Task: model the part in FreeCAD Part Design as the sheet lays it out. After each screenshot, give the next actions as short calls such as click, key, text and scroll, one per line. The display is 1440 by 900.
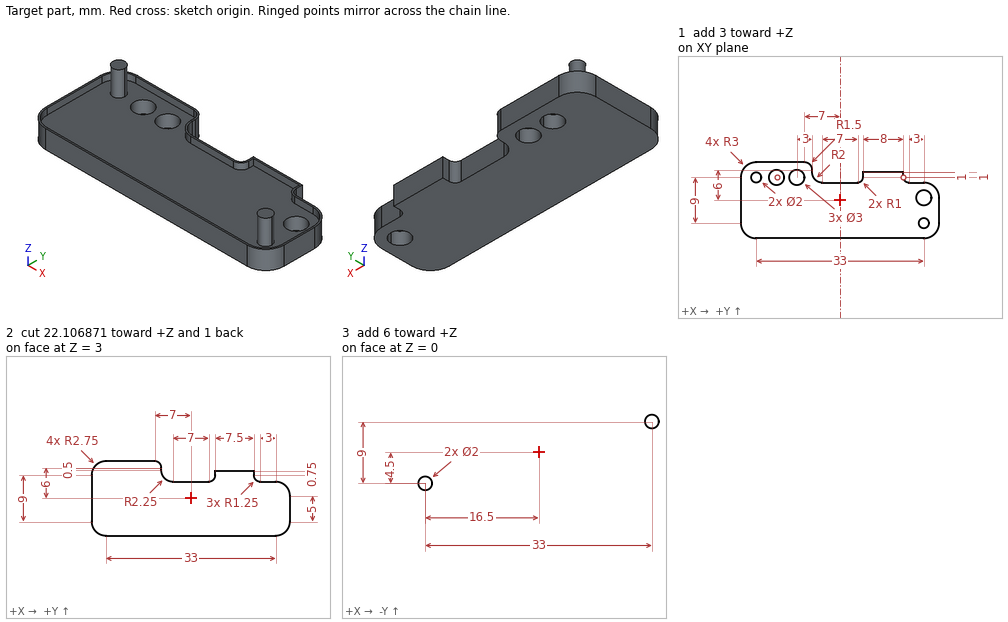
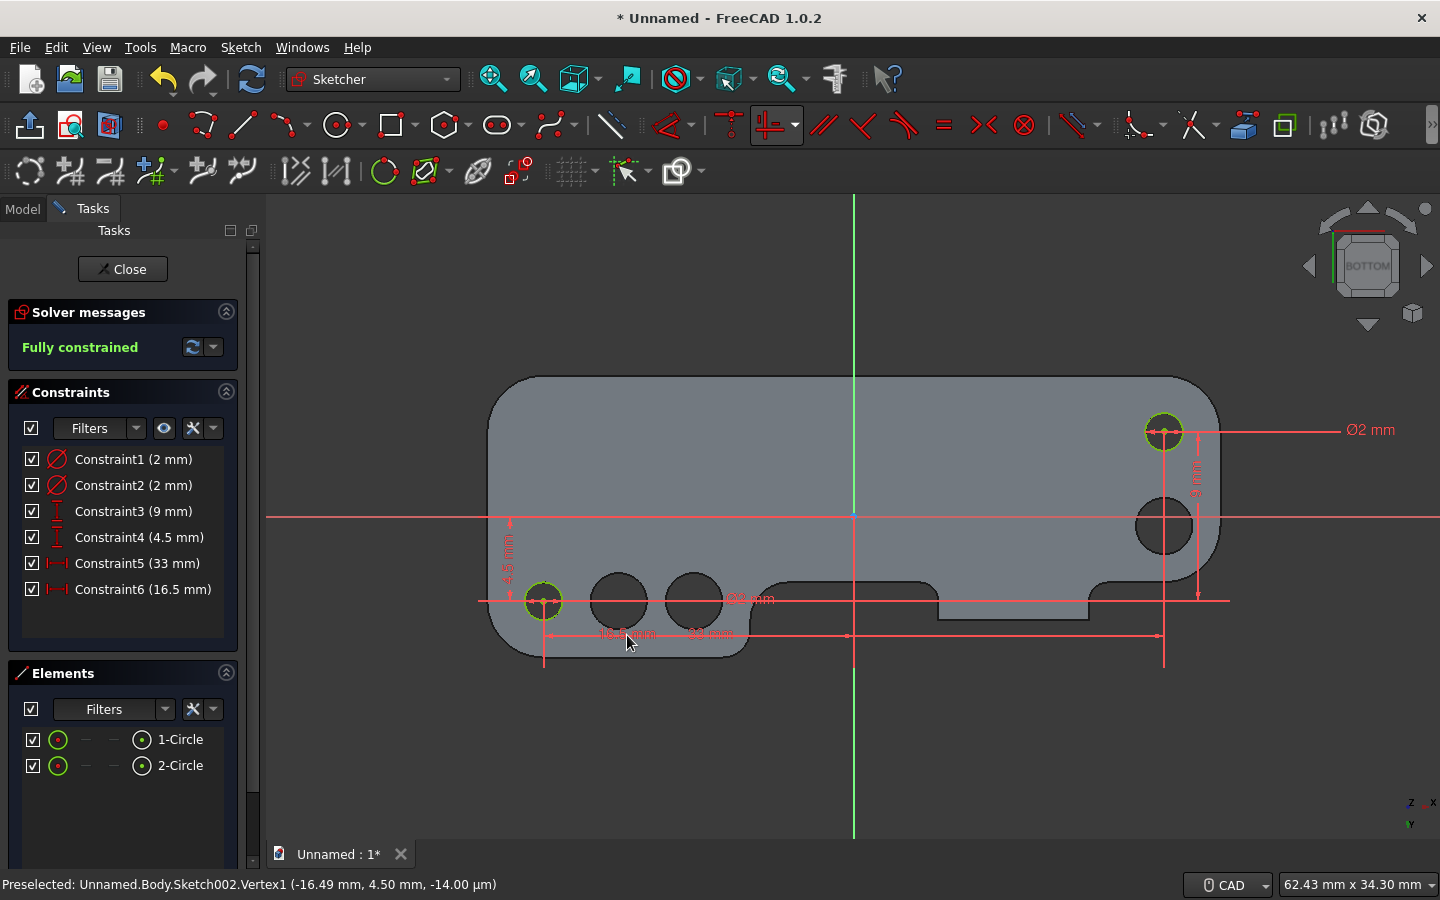
click(123, 269)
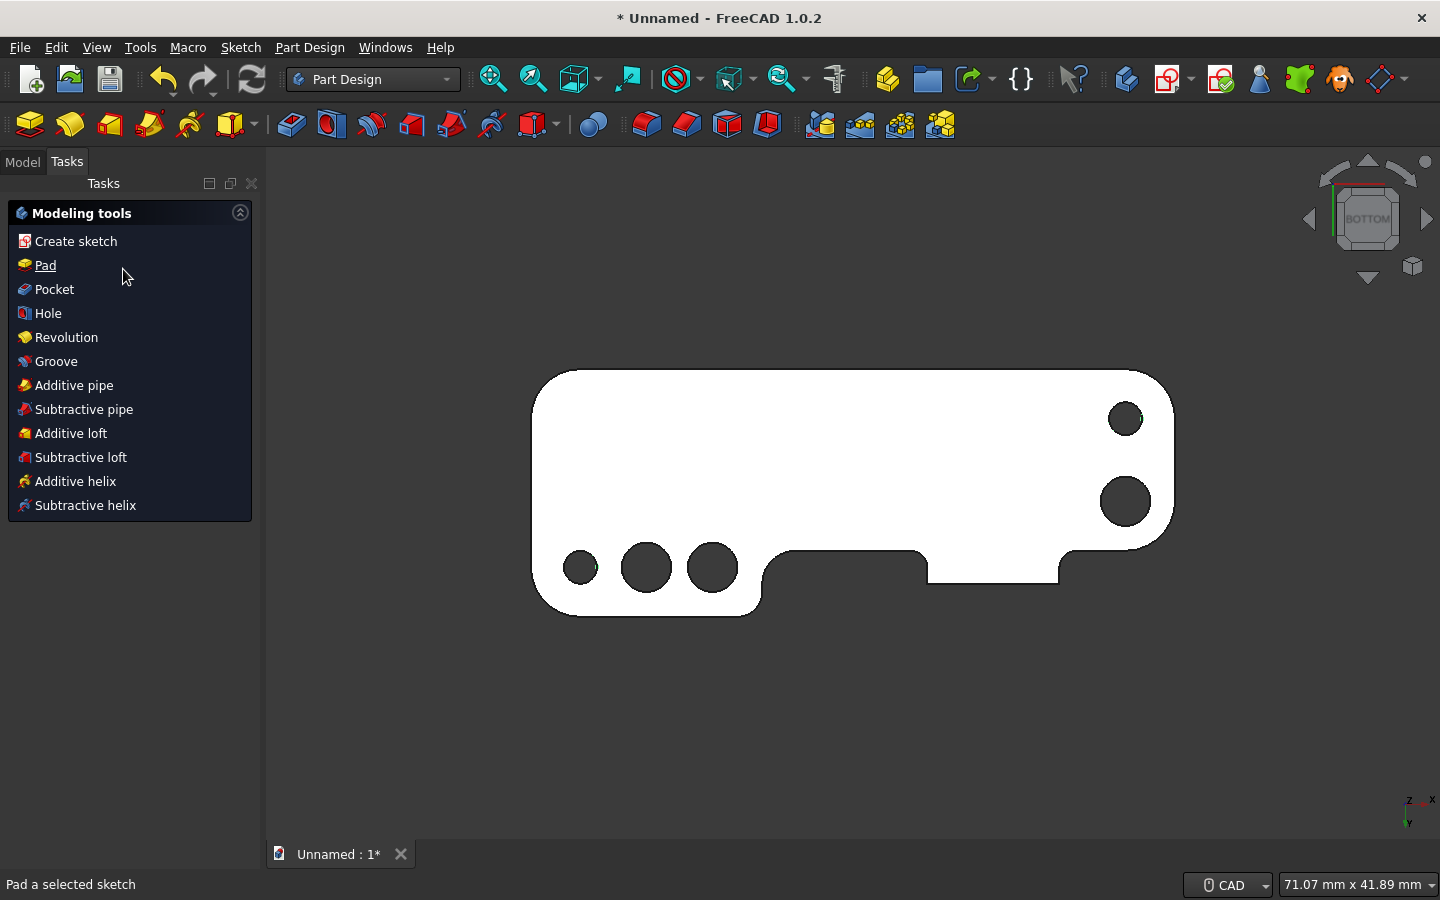
click(30, 124)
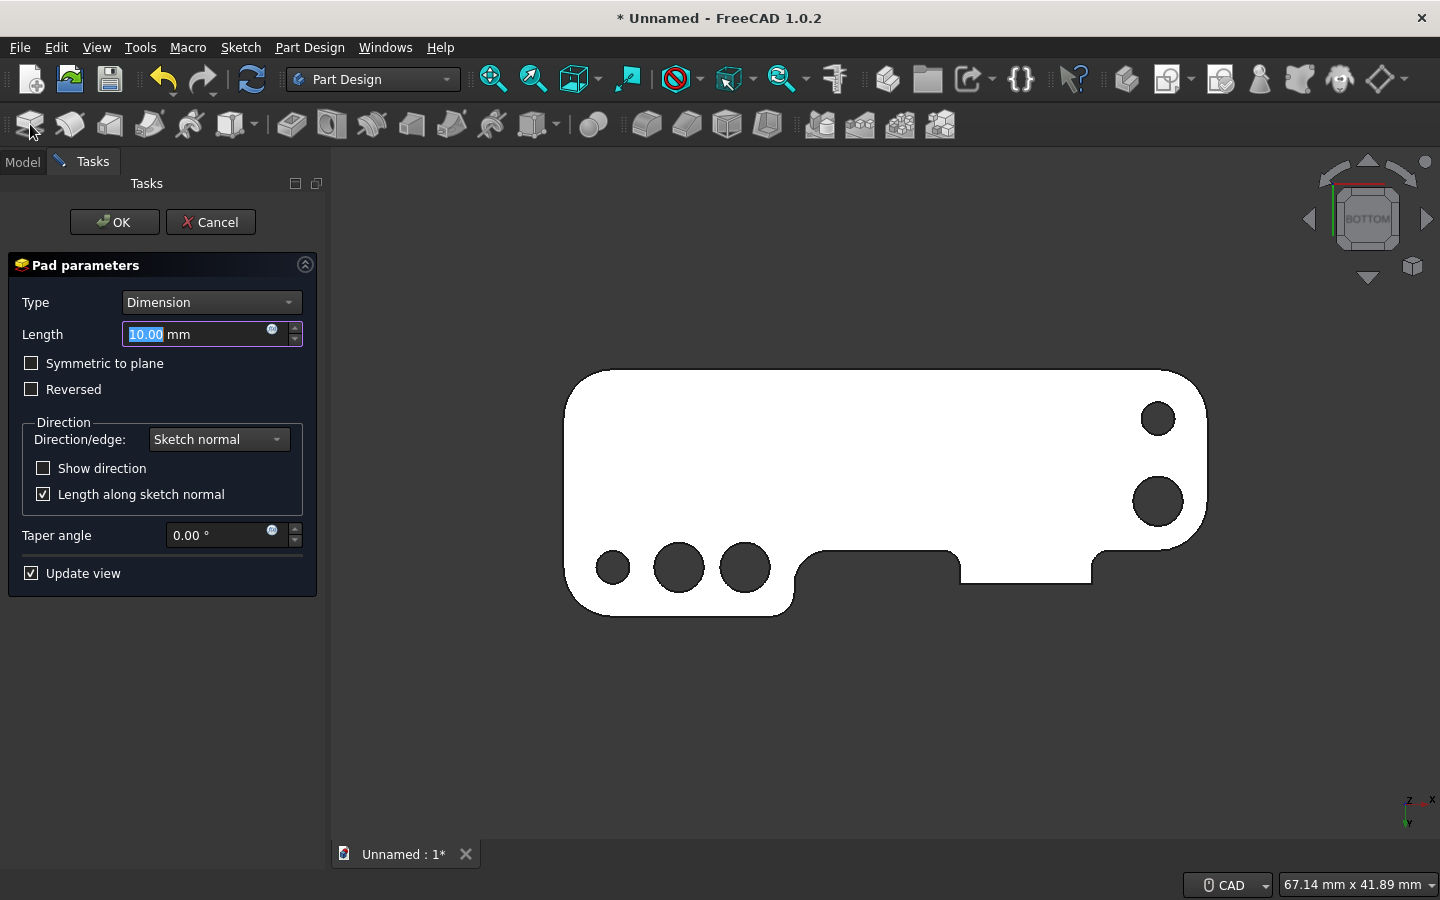
text(6)
key(Tab)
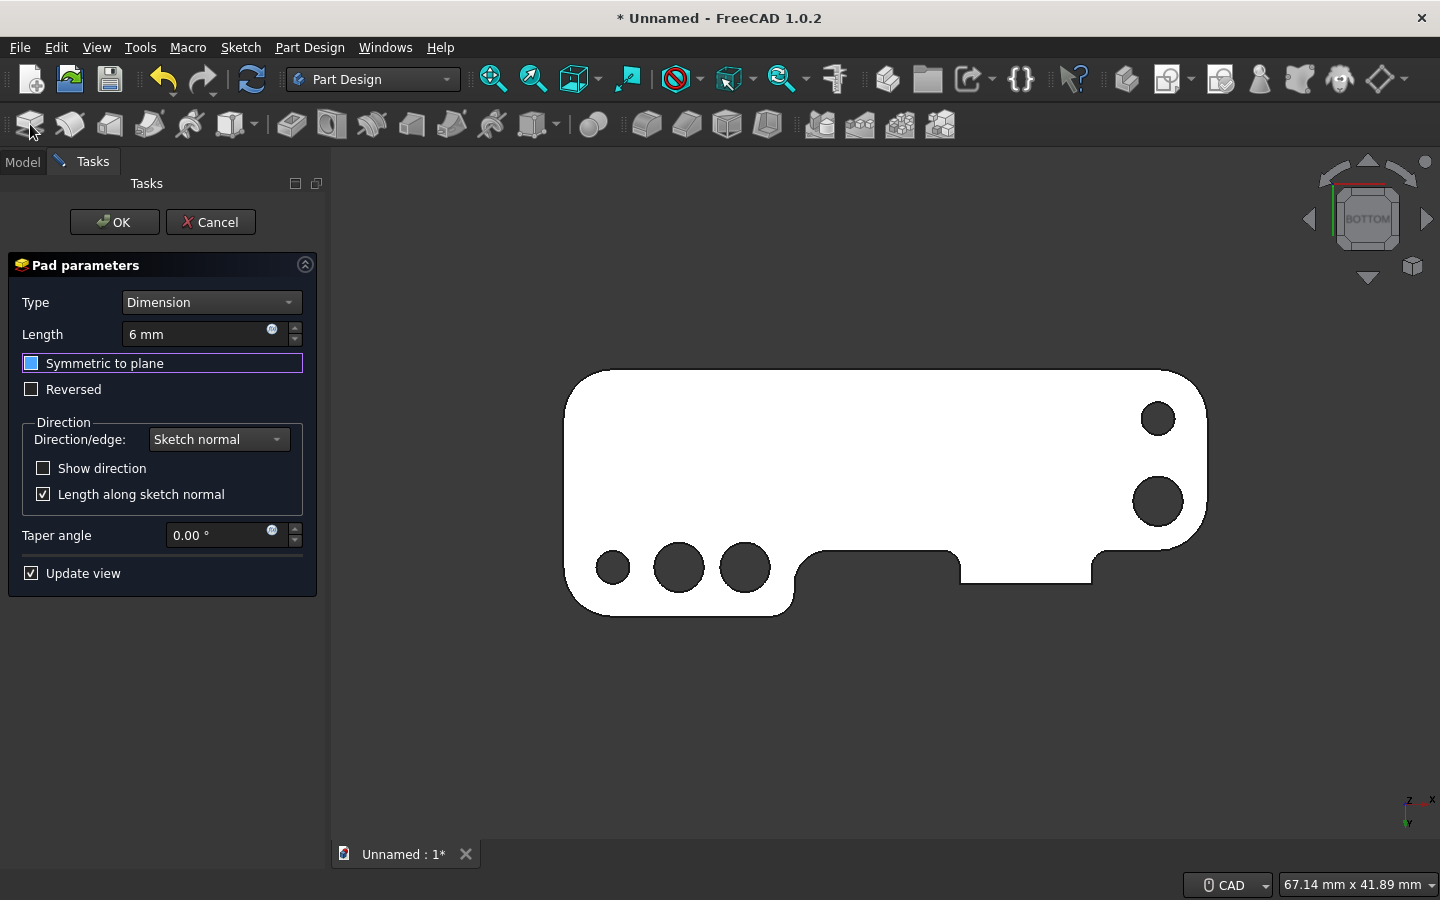
click(30, 389)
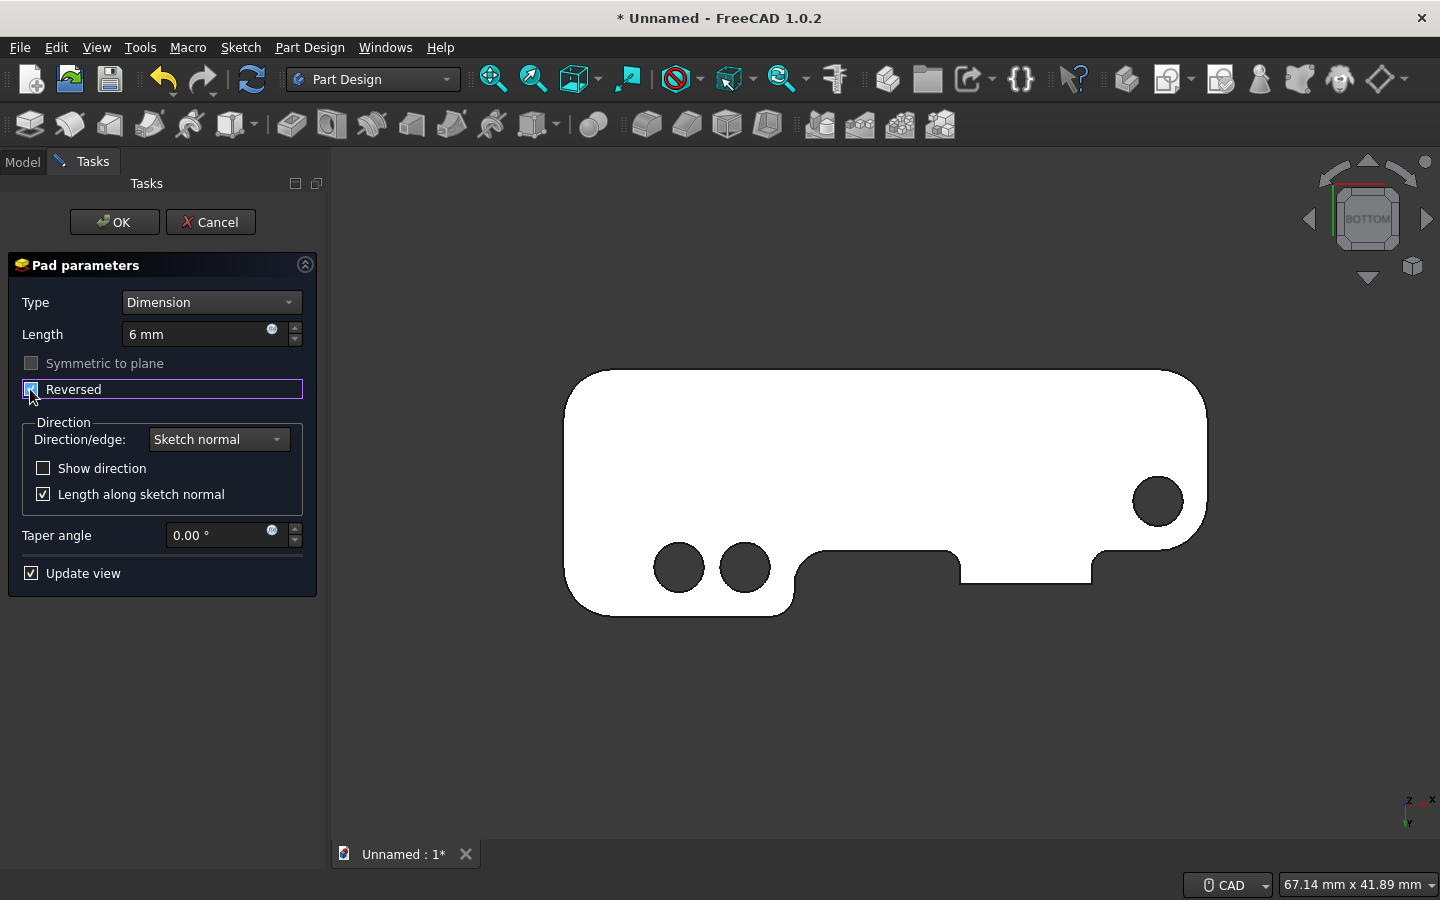
click(115, 222)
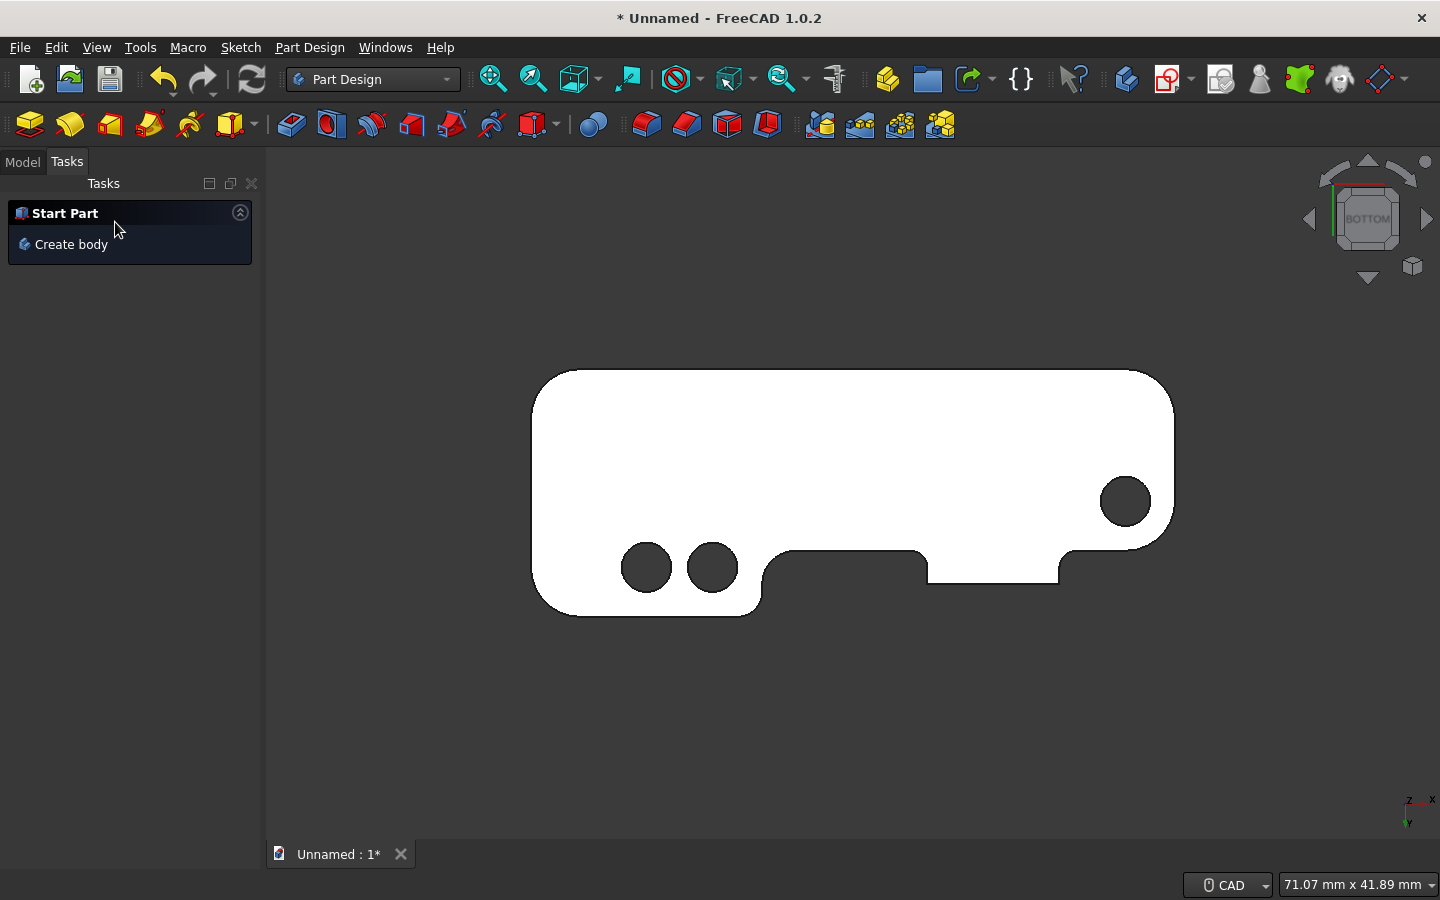
key(0)